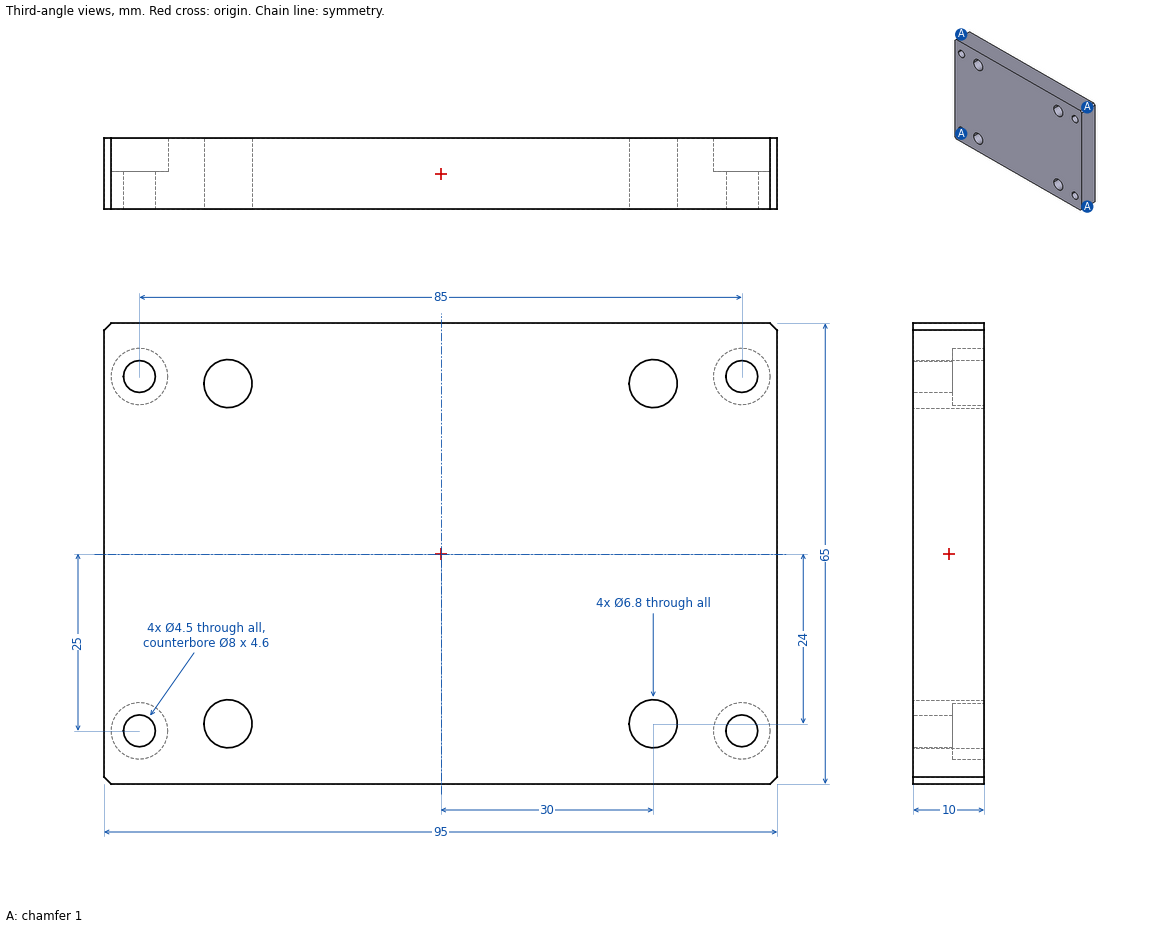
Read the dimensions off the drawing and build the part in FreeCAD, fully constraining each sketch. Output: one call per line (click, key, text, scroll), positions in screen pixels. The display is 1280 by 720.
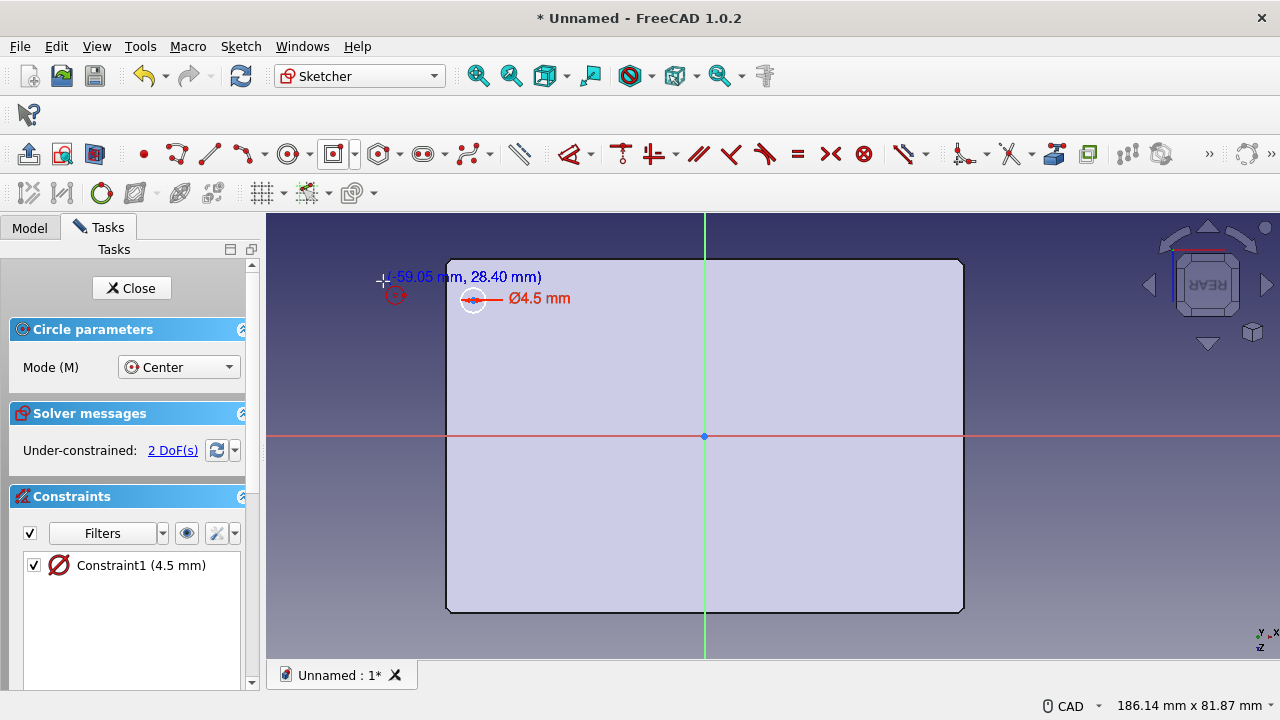
scroll(473, 572, up, 4)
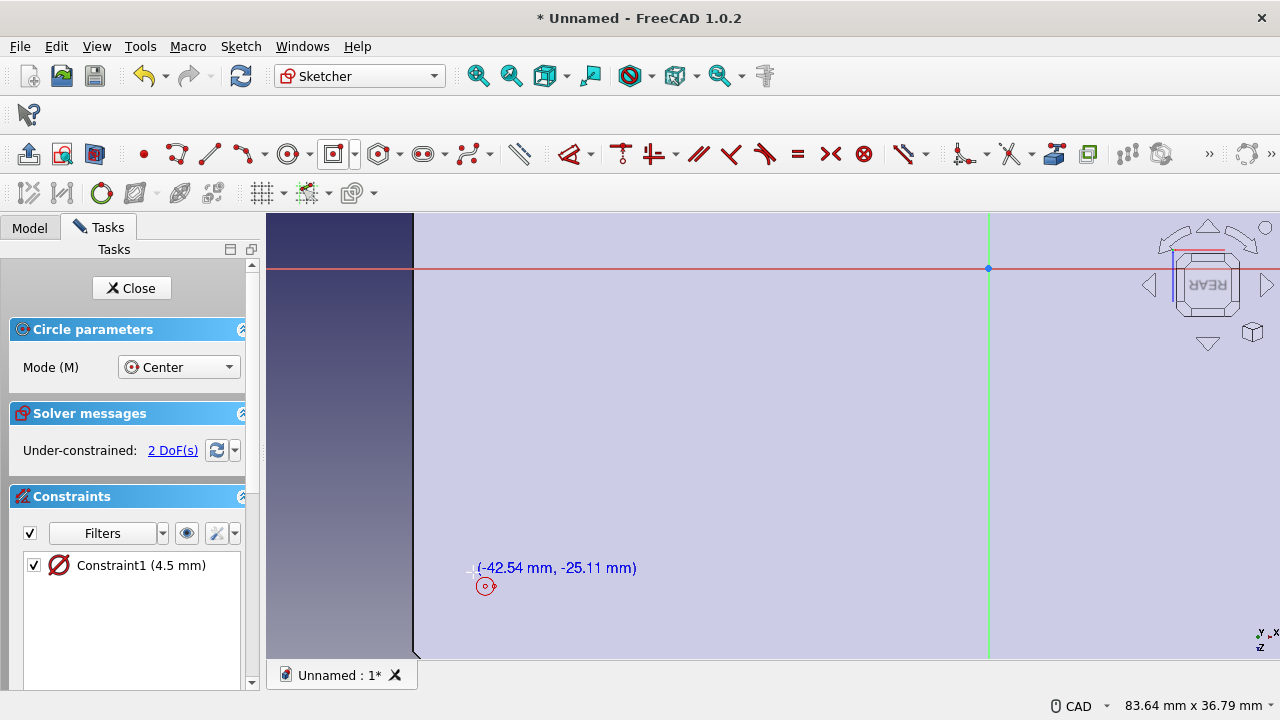
click(473, 572)
move(493, 553)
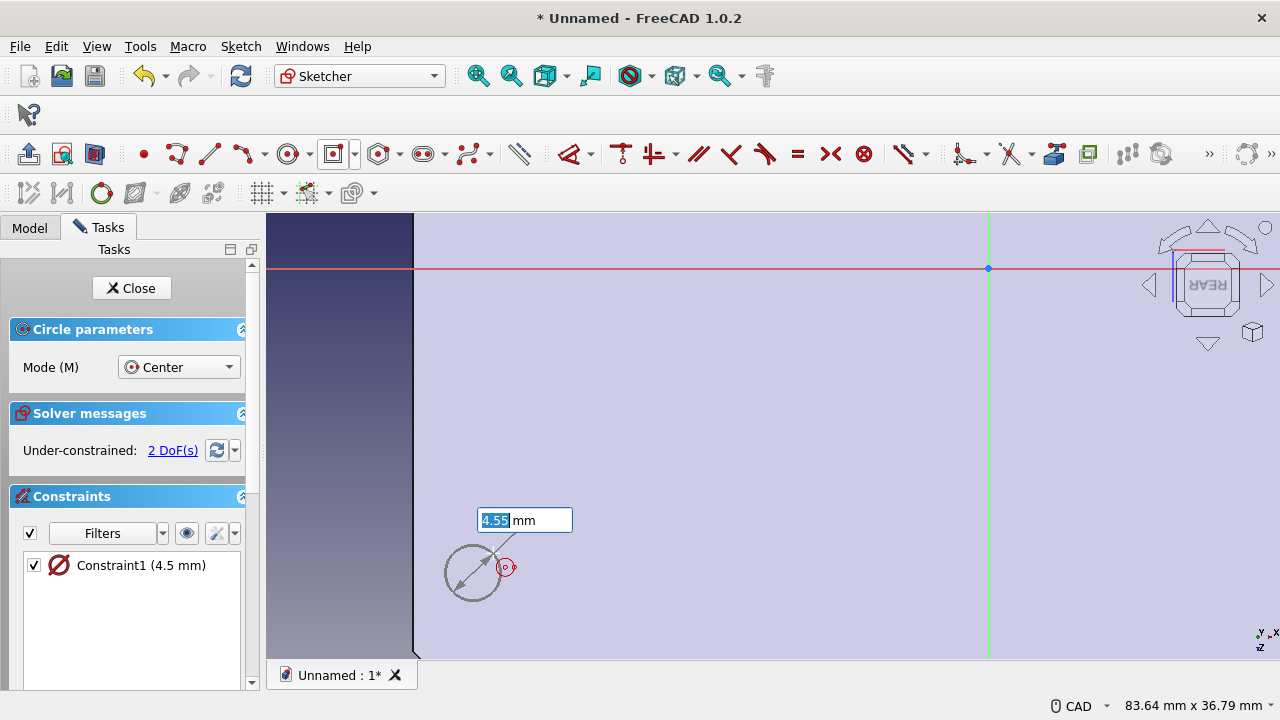
text(4.5)
key(Return)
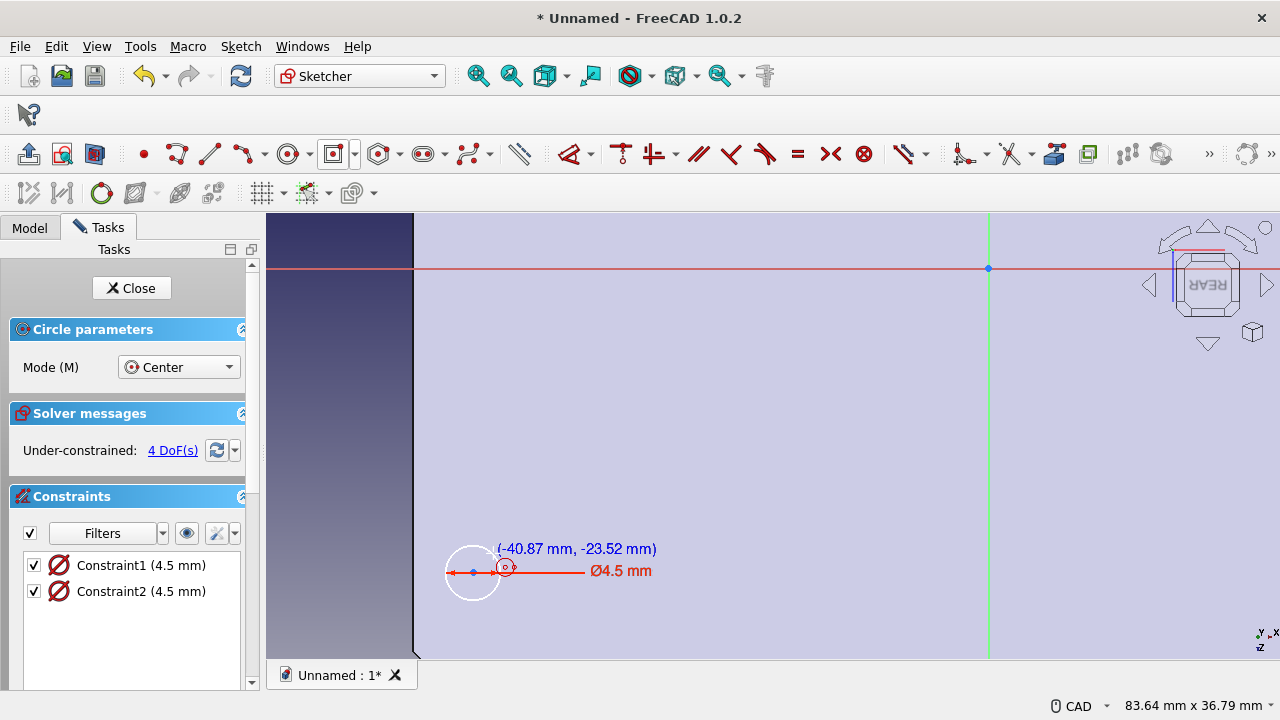
scroll(473, 572, down, 4)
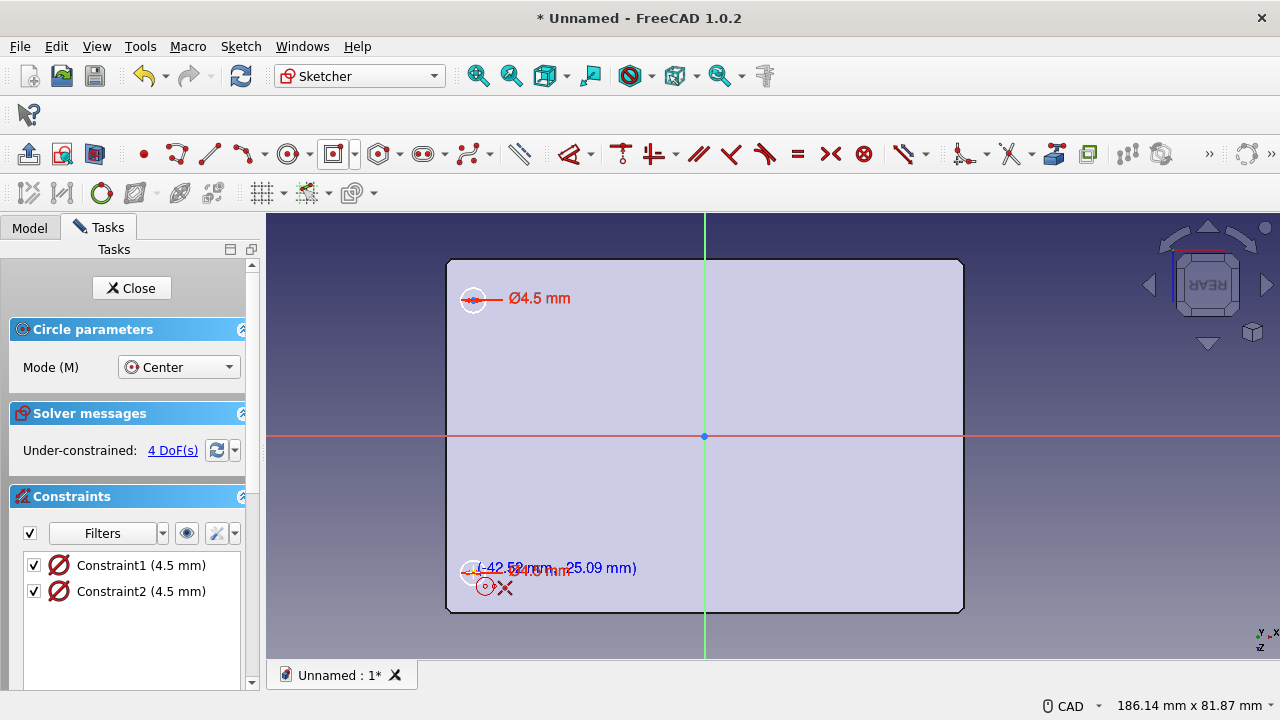
scroll(936, 572, up, 4)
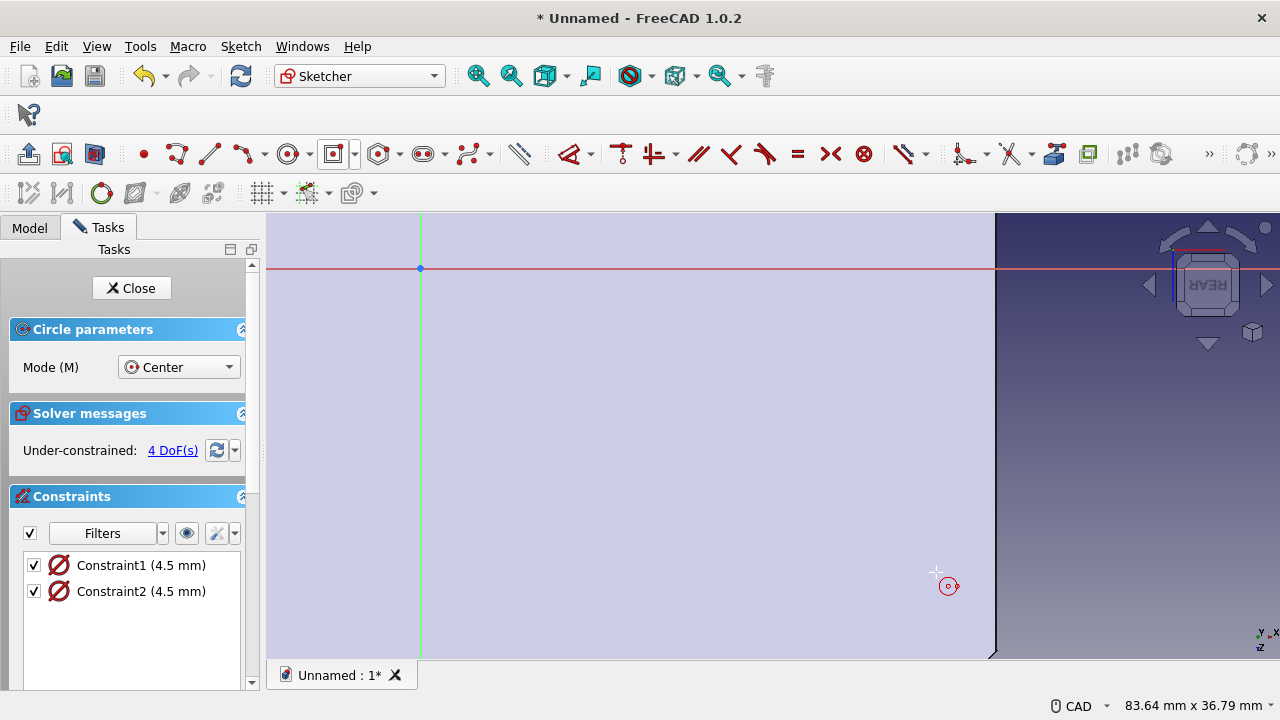
click(936, 572)
move(955, 553)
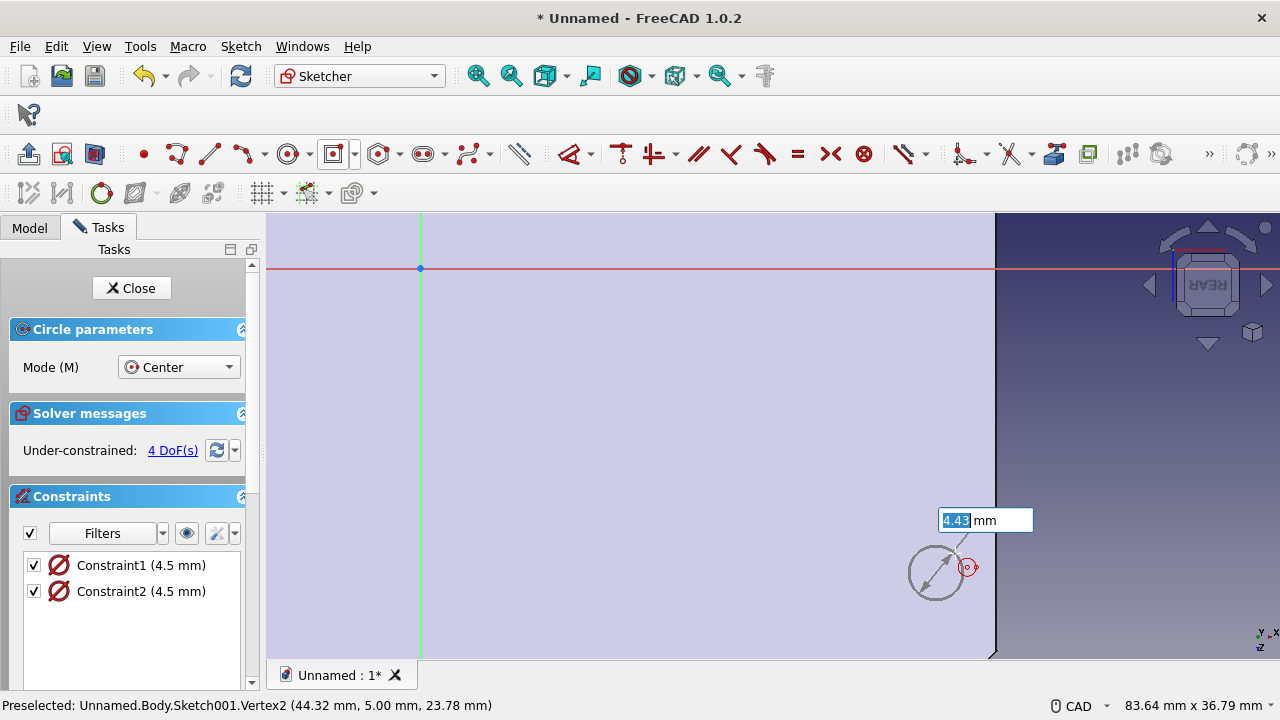
text(4.5)
key(Return)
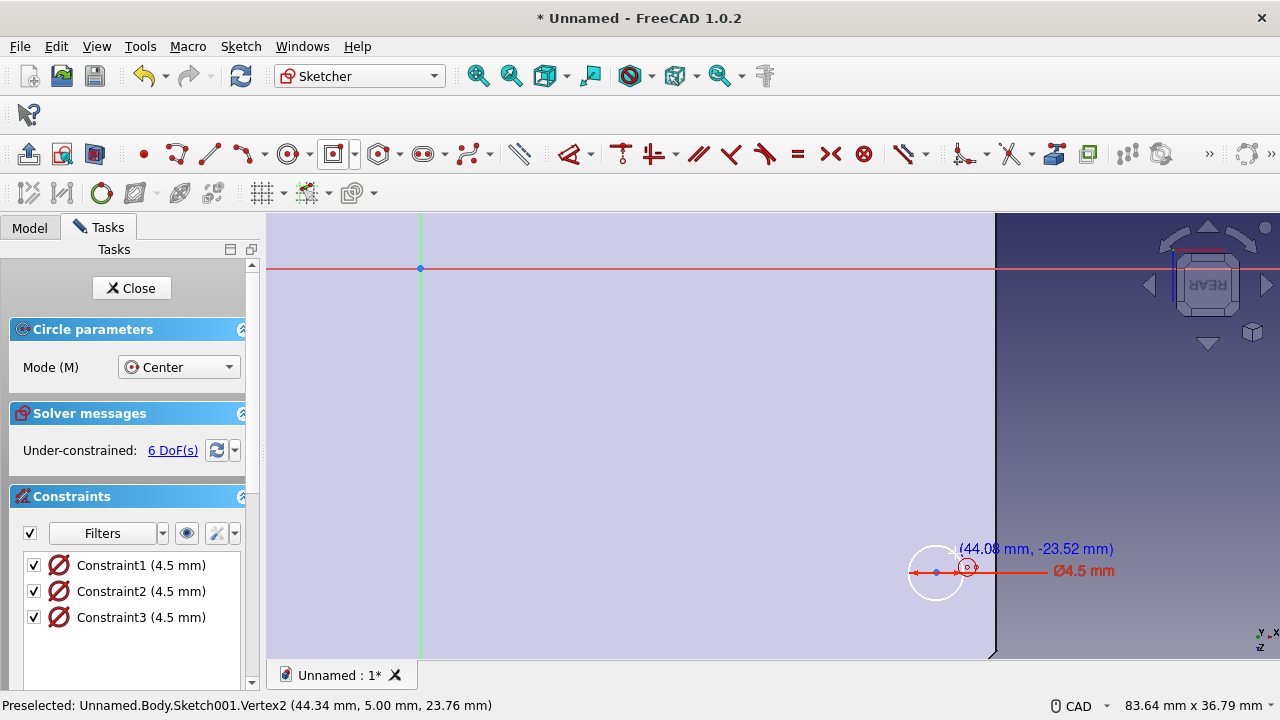
scroll(936, 572, down, 4)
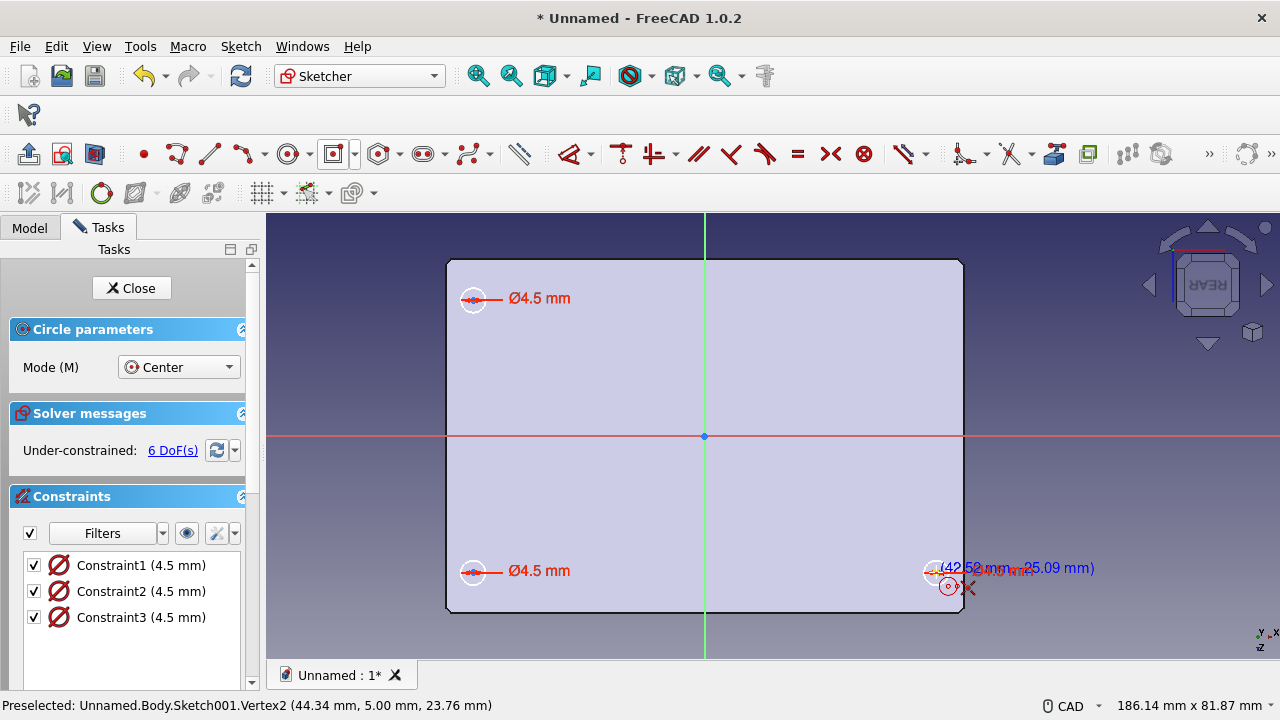
scroll(936, 300, up, 4)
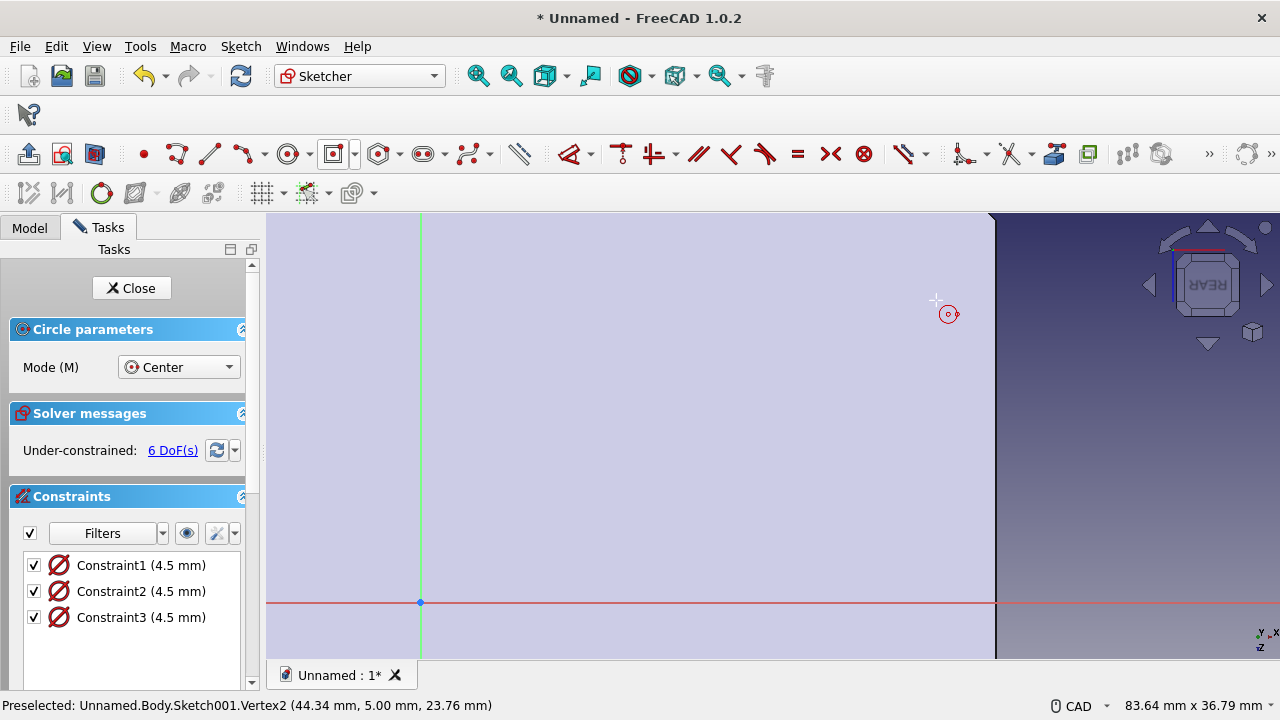
click(936, 300)
move(955, 281)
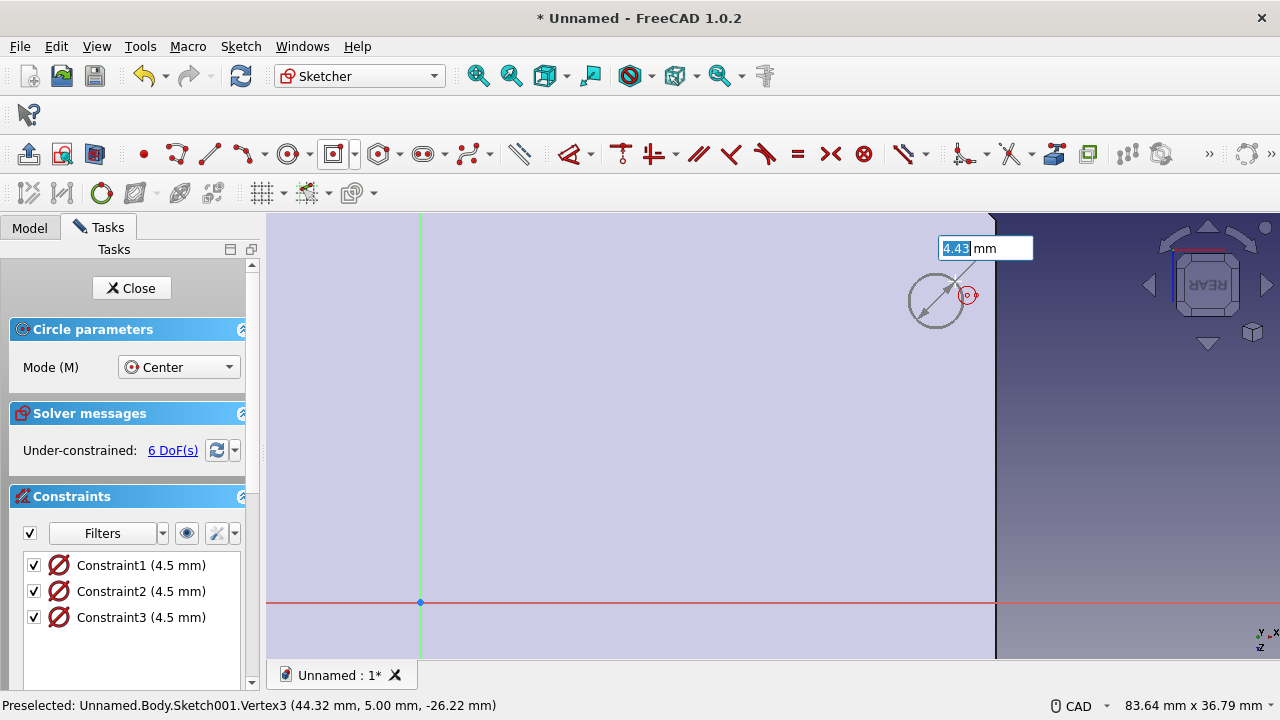
text(4.5)
key(Return)
key(Escape)